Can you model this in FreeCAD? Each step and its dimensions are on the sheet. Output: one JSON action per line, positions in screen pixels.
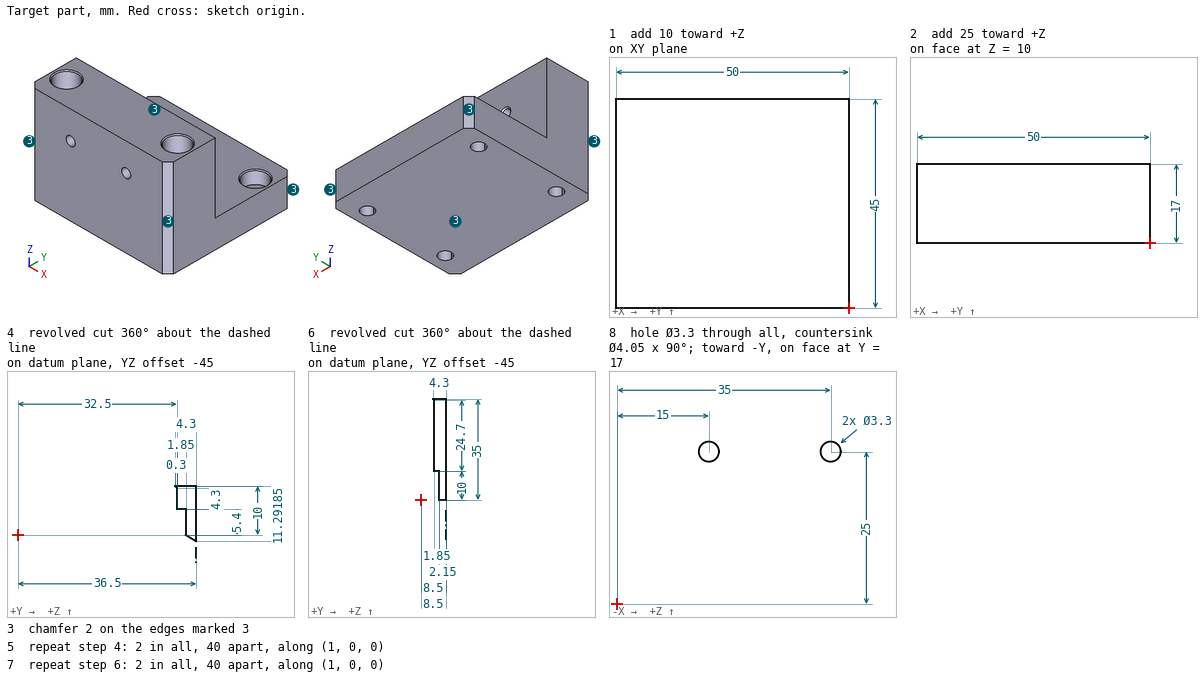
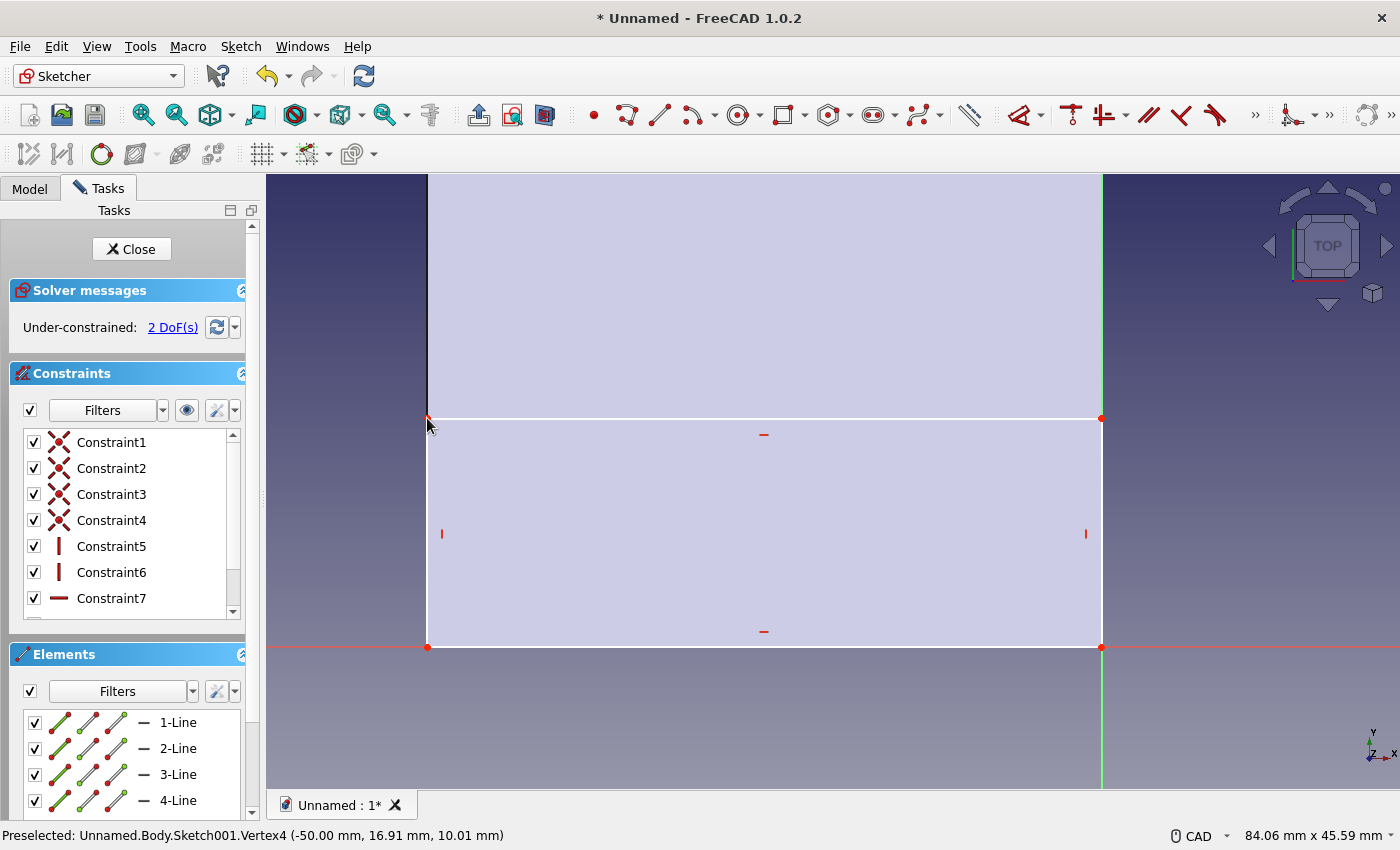
{"action": "left_click", "coordinate": [1102, 579]}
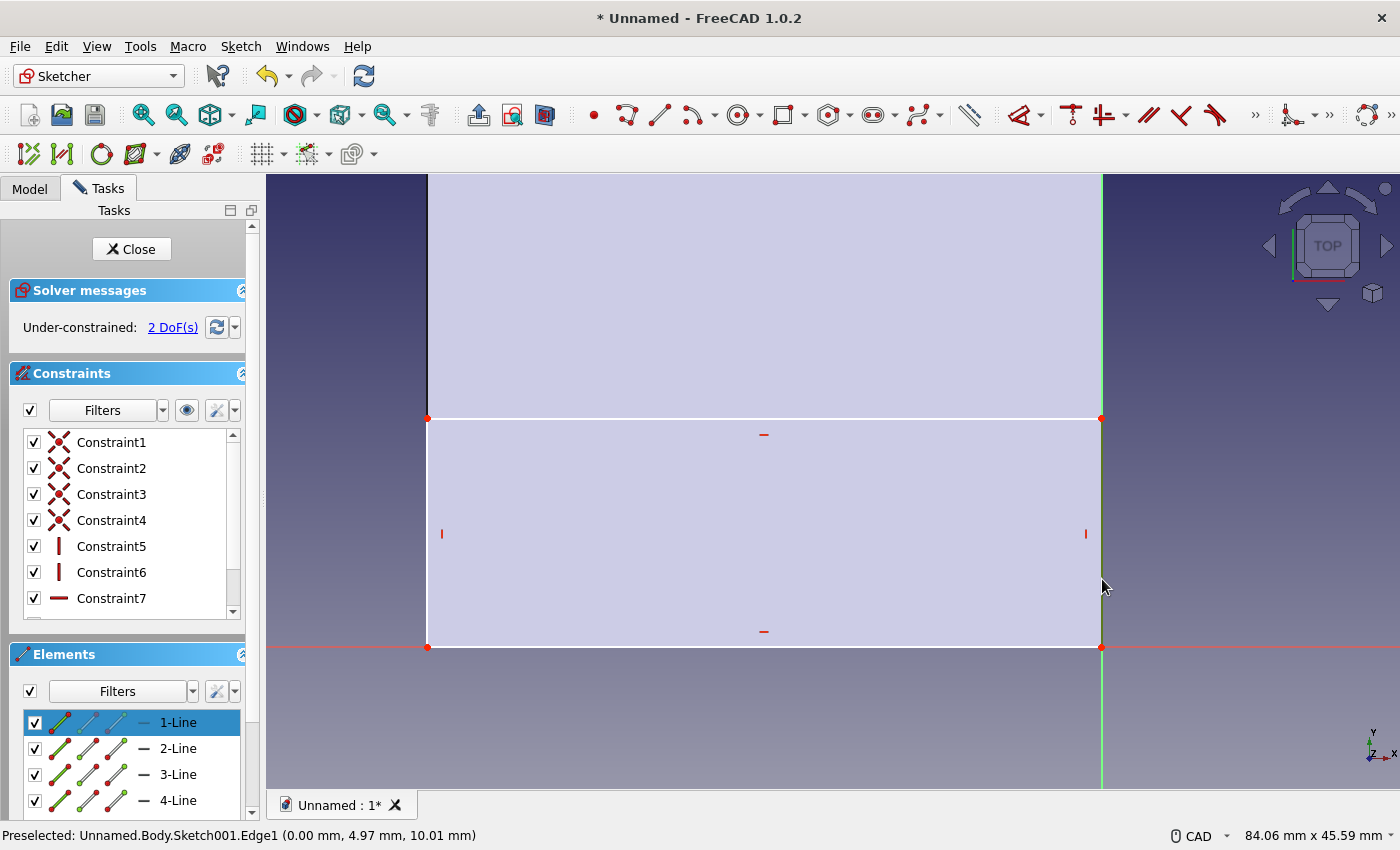
{"action": "key", "text": "i"}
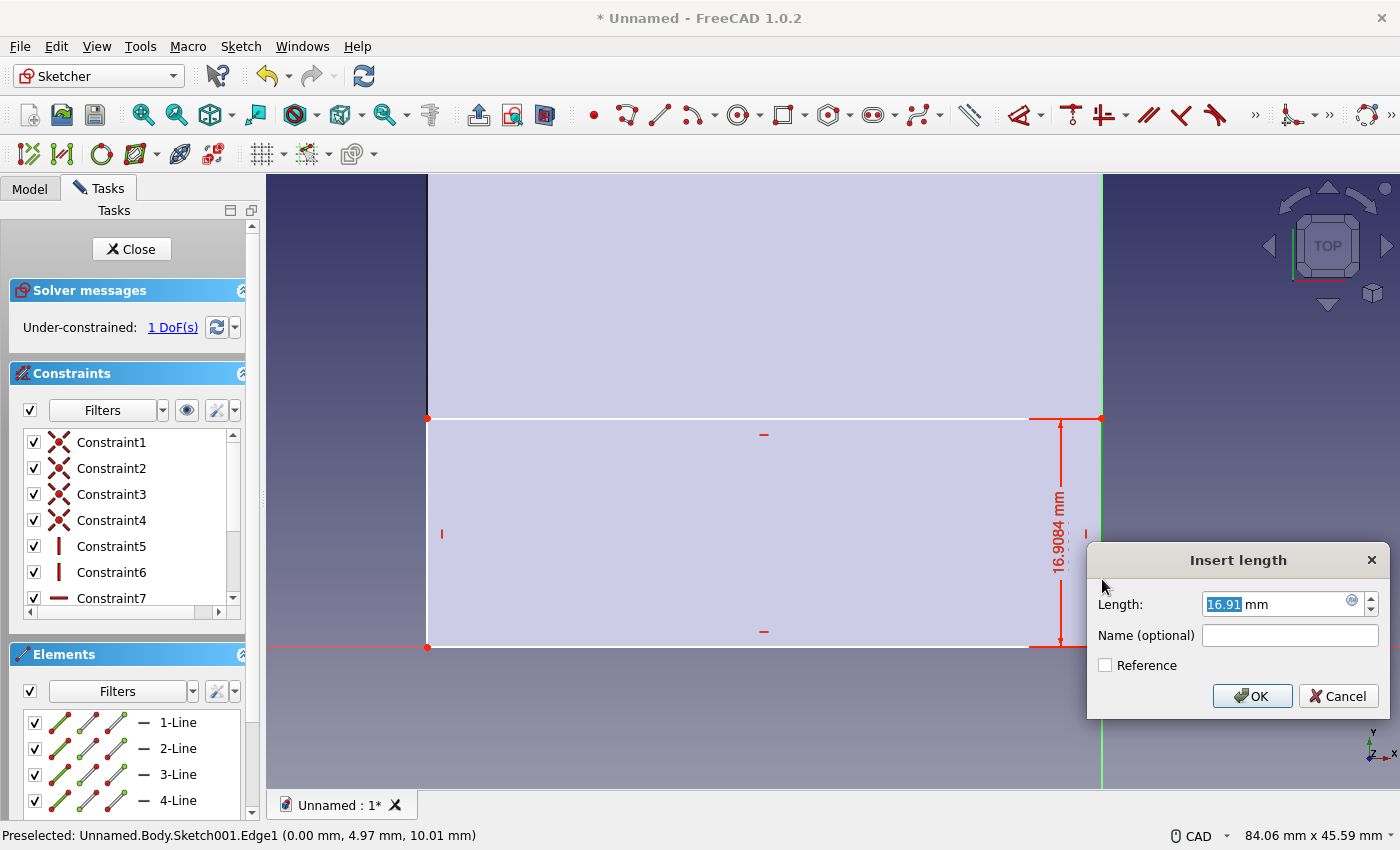
{"action": "type", "text": "17"}
{"action": "key", "text": "Return"}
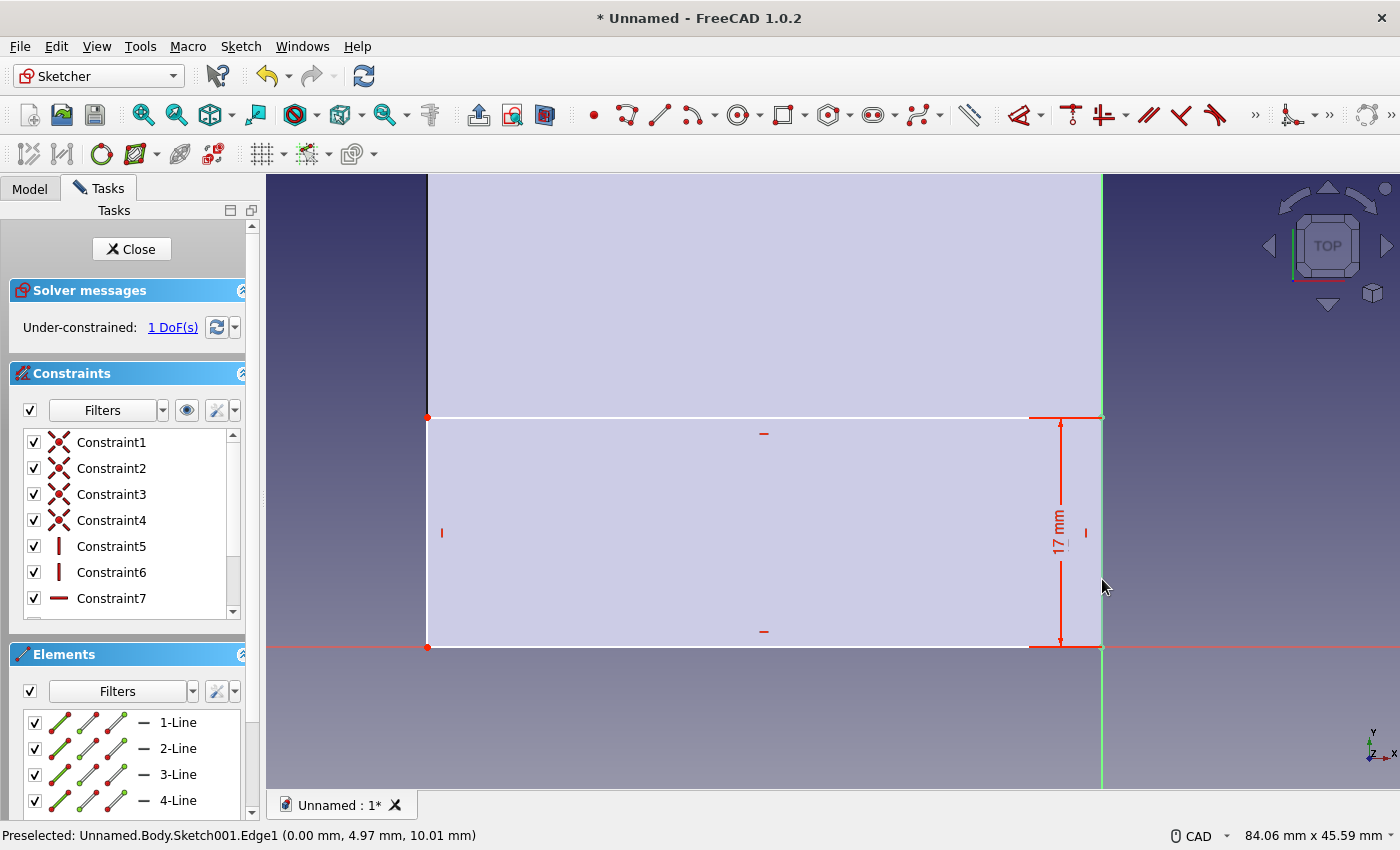
{"action": "left_click", "coordinate": [899, 418]}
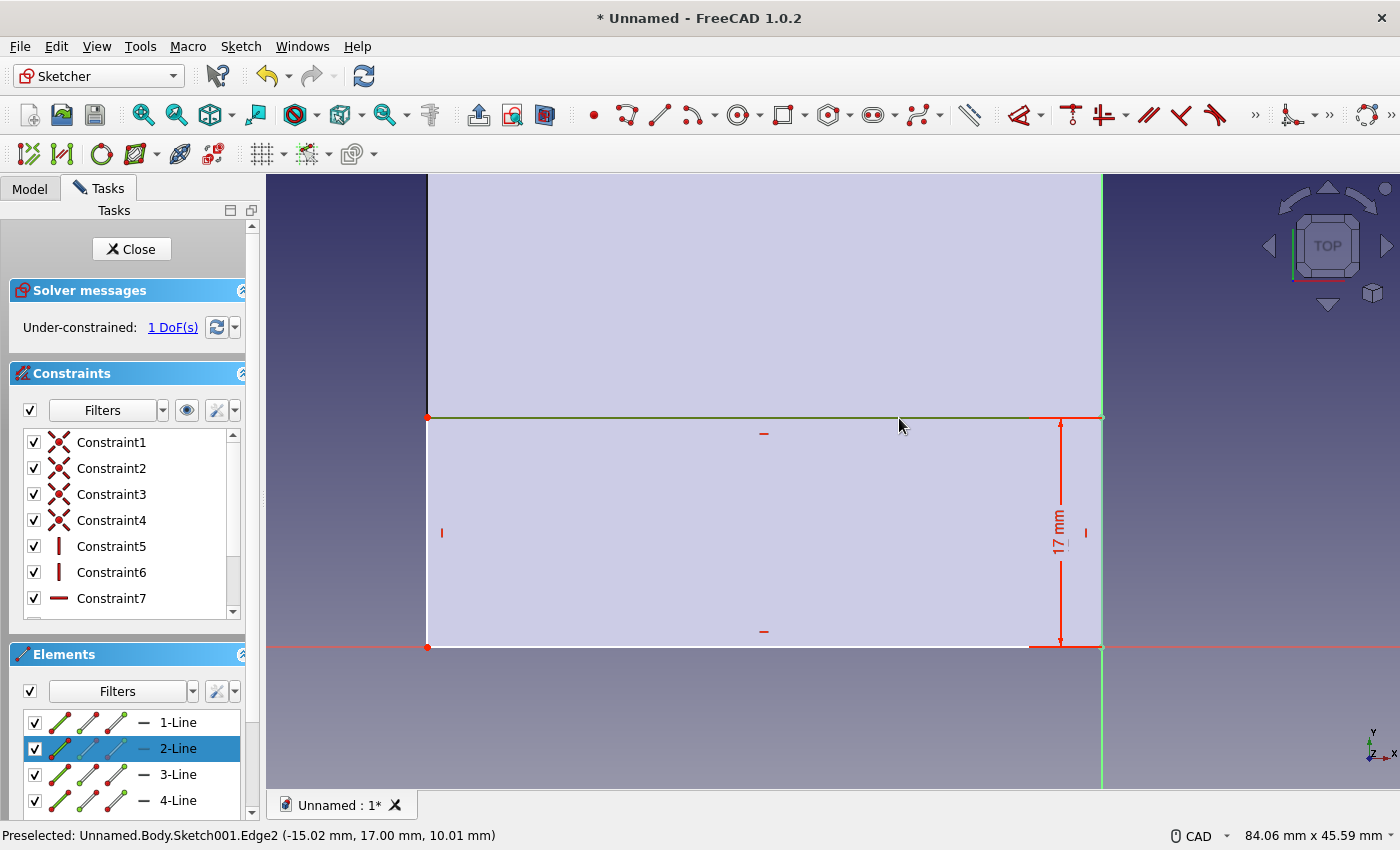
{"action": "key", "text": "l"}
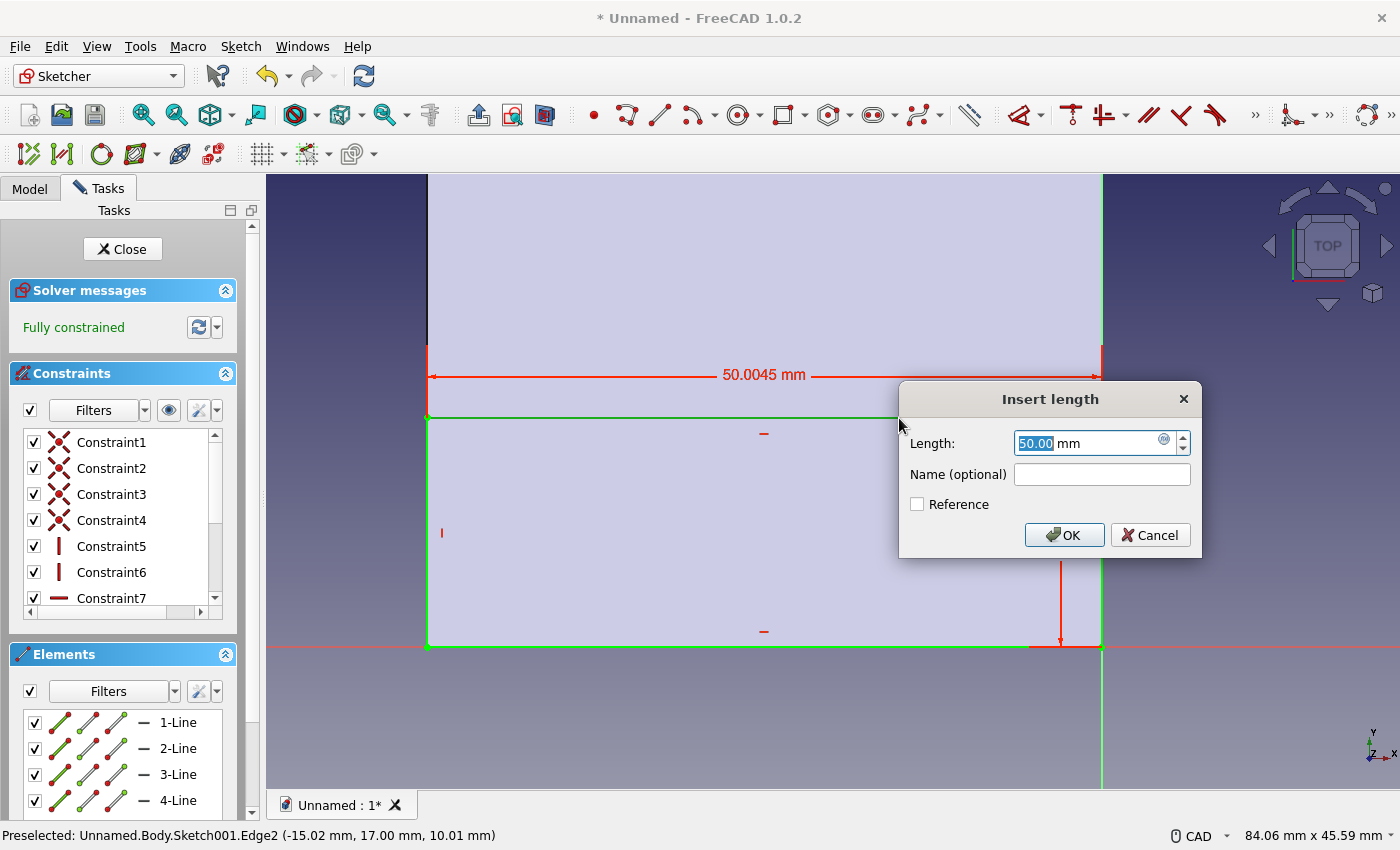
{"action": "type", "text": "50"}
{"action": "key", "text": "Return"}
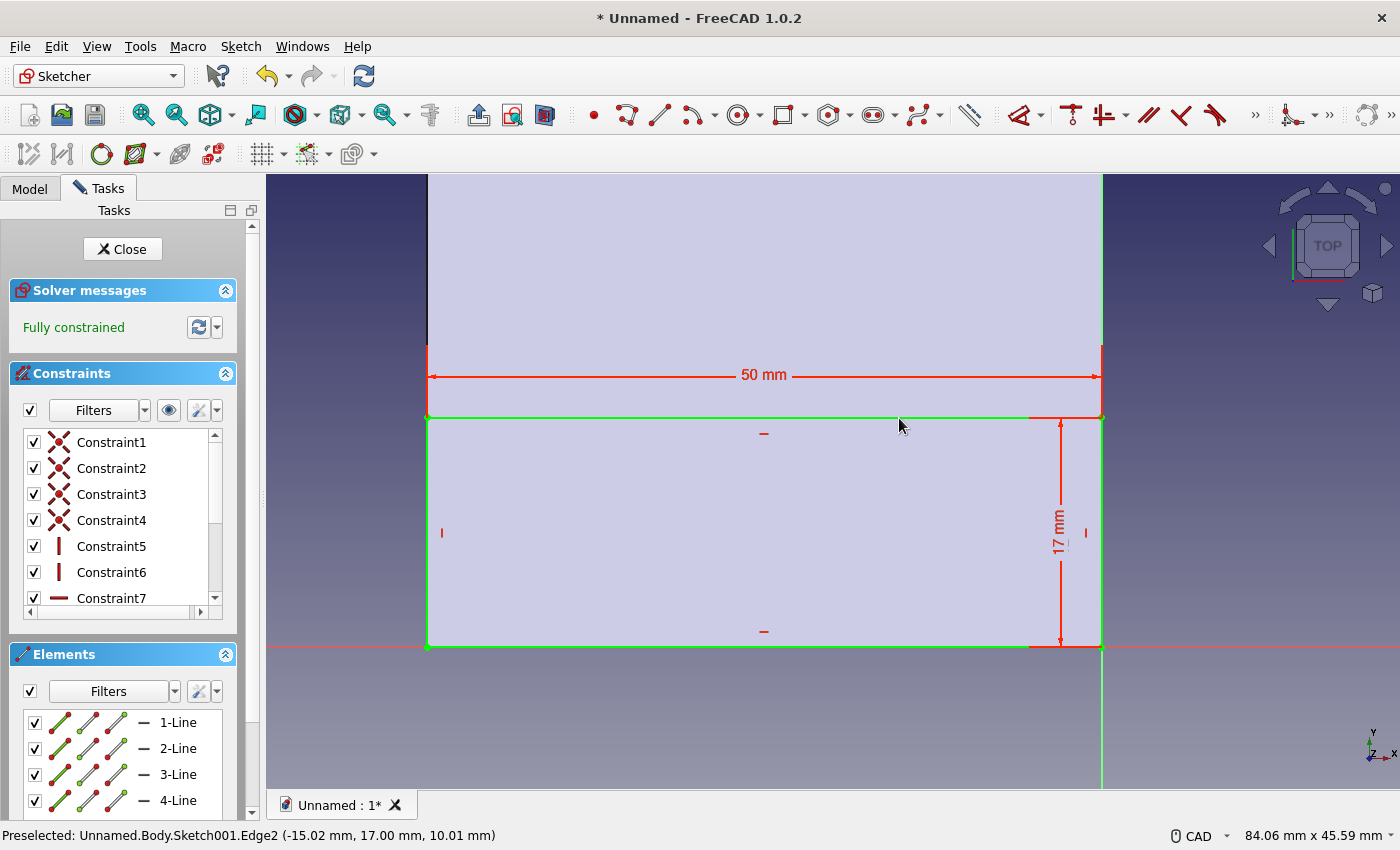
{"action": "left_click", "coordinate": [123, 249]}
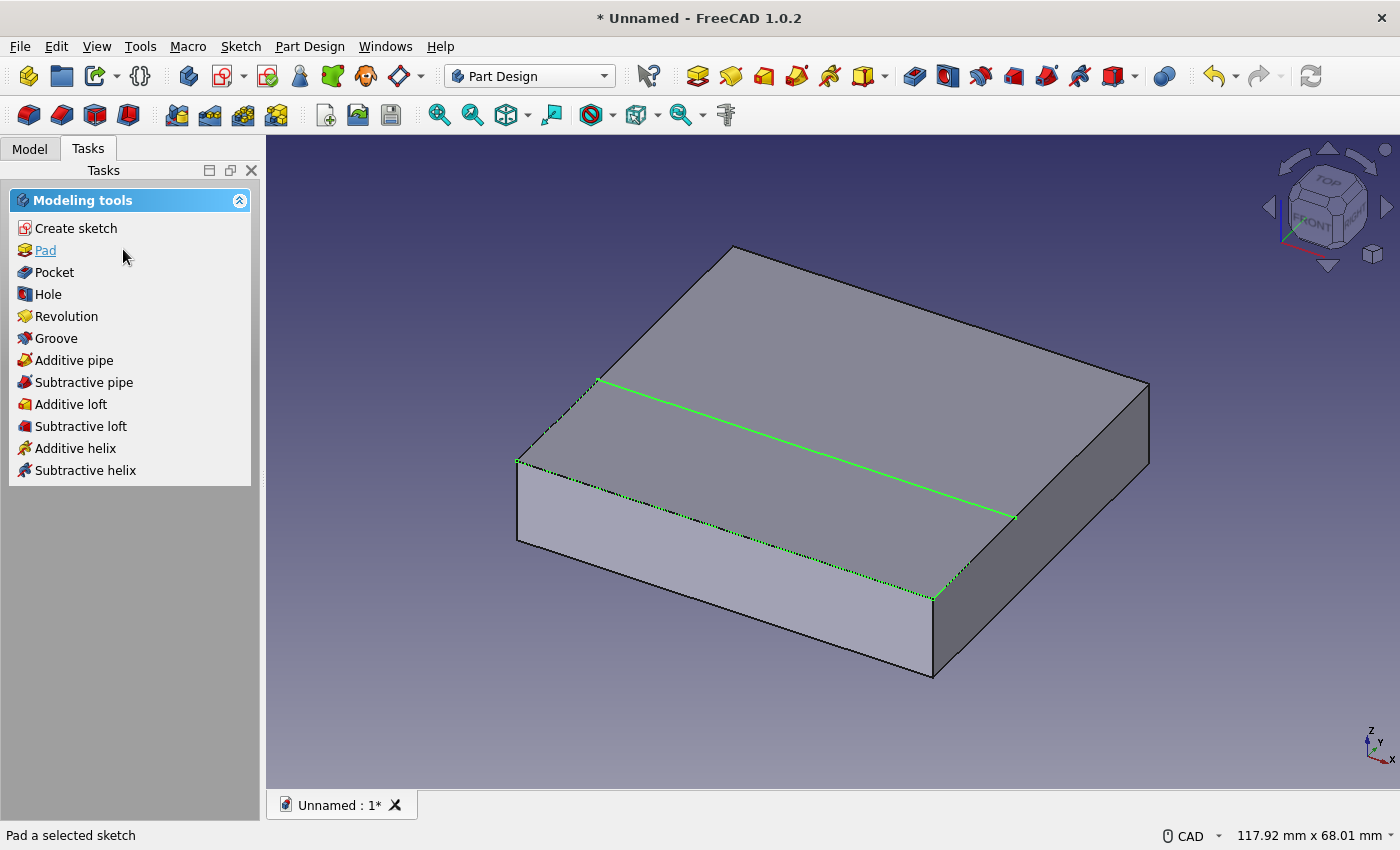
{"action": "left_click", "coordinate": [698, 76]}